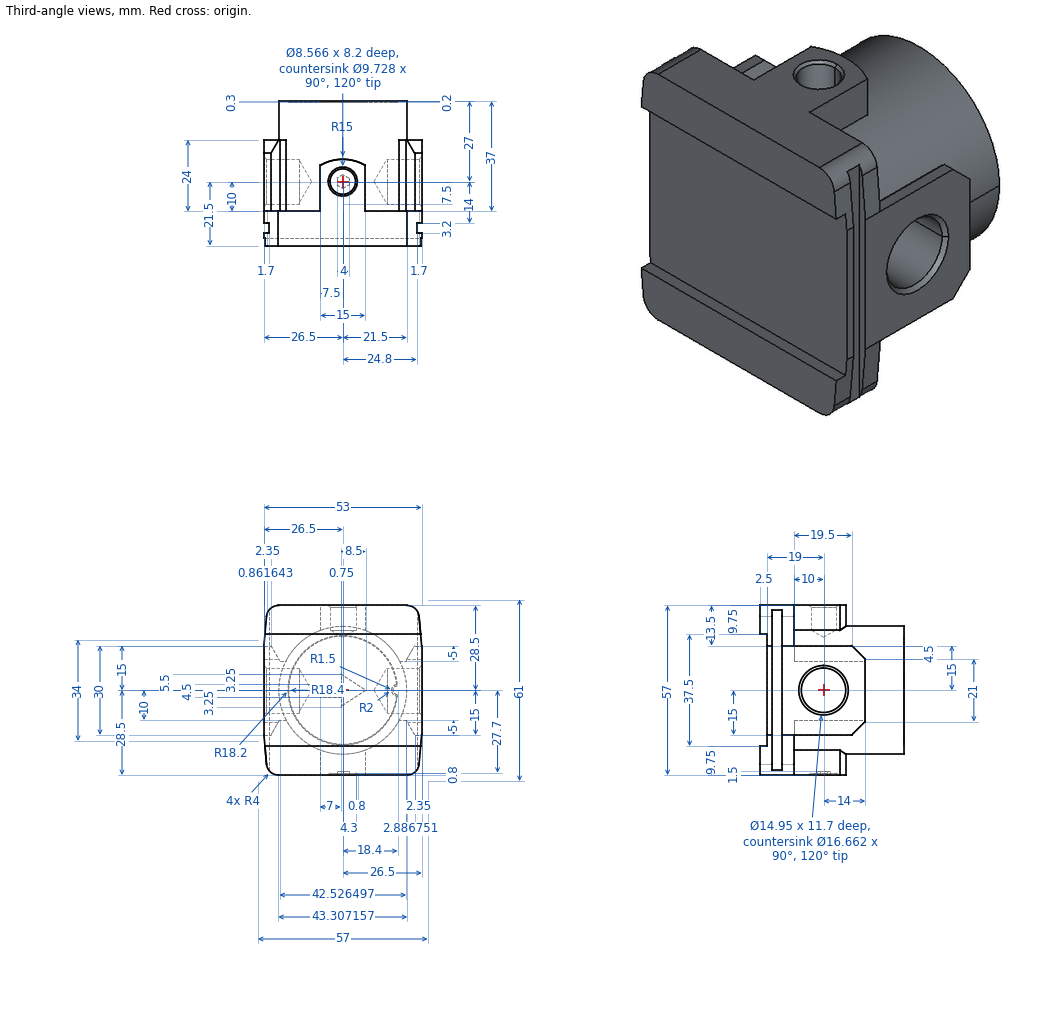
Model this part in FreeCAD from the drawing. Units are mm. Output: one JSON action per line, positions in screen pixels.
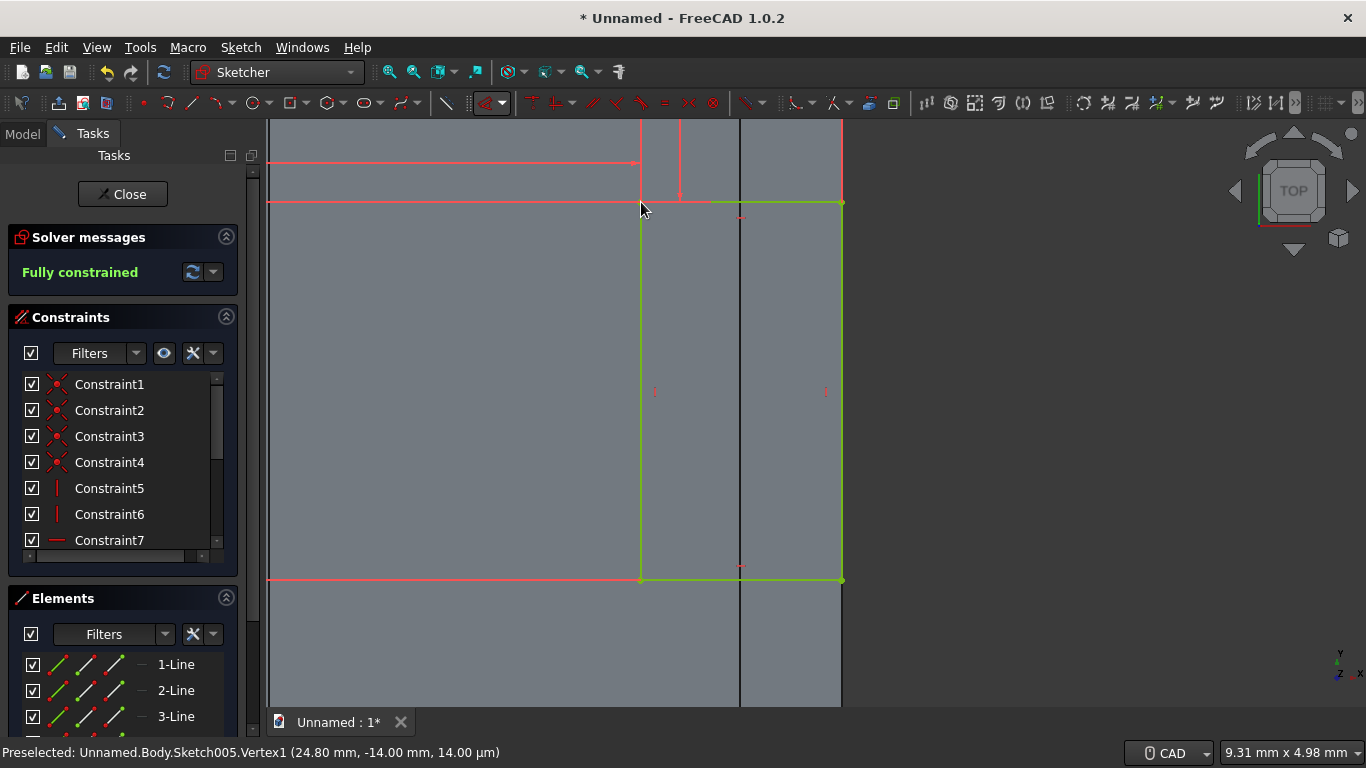
{"action": "left_click", "coordinate": [123, 194]}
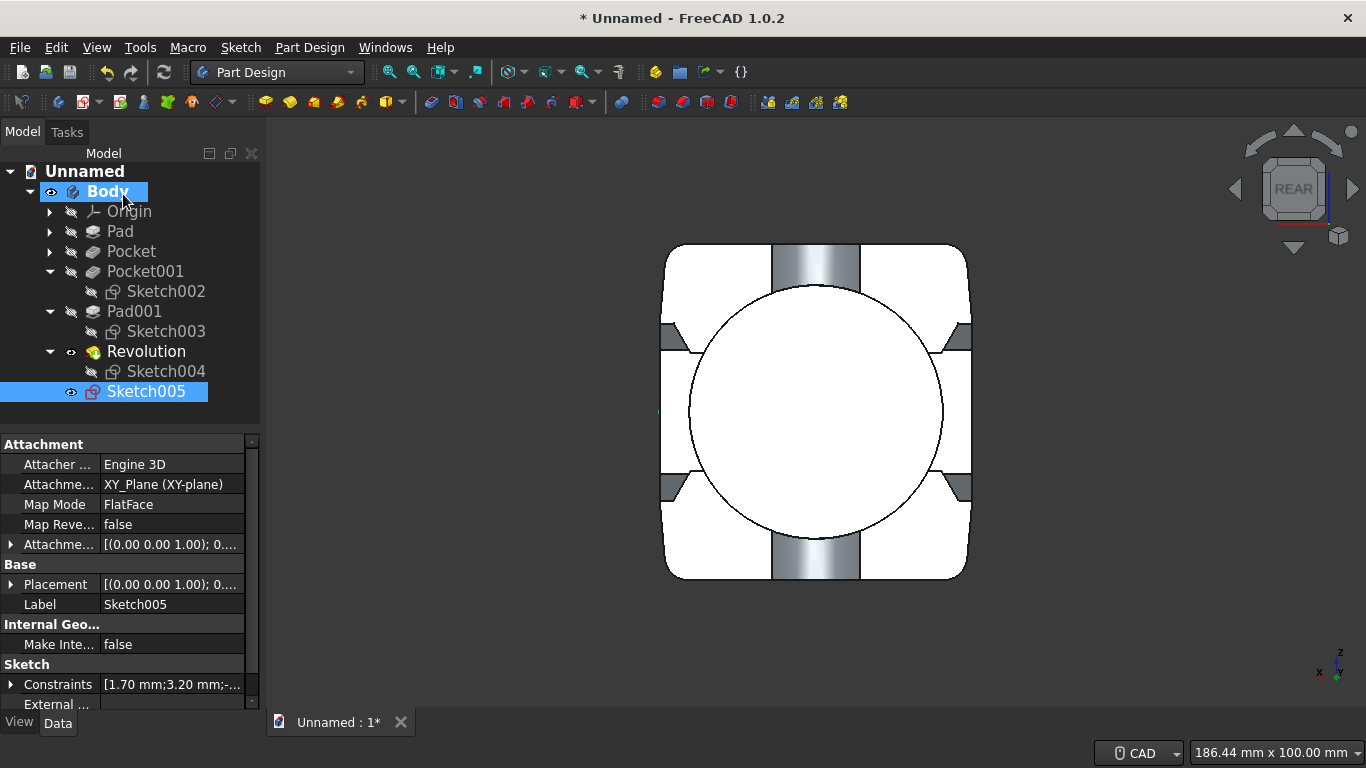
{"action": "left_click", "coordinate": [432, 102]}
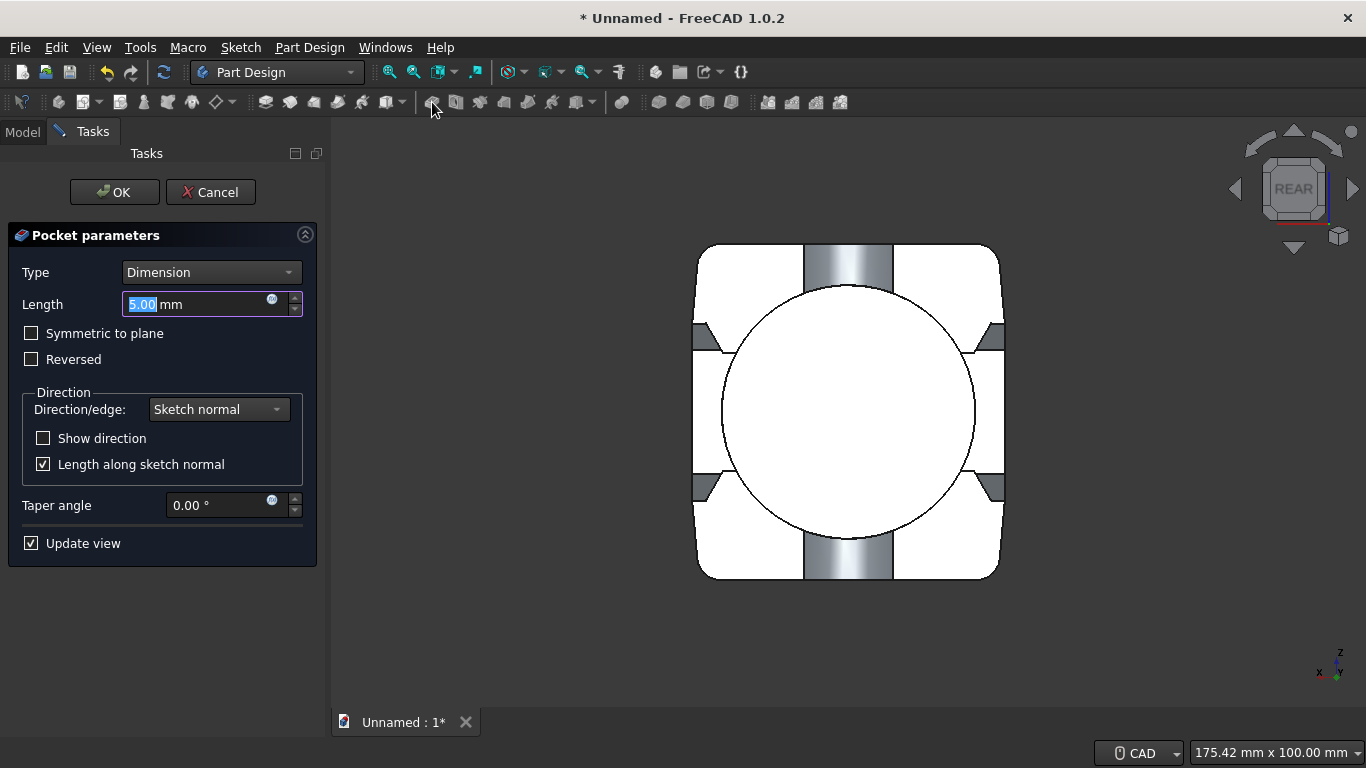
{"action": "type", "text": "57"}
{"action": "key", "text": "Tab"}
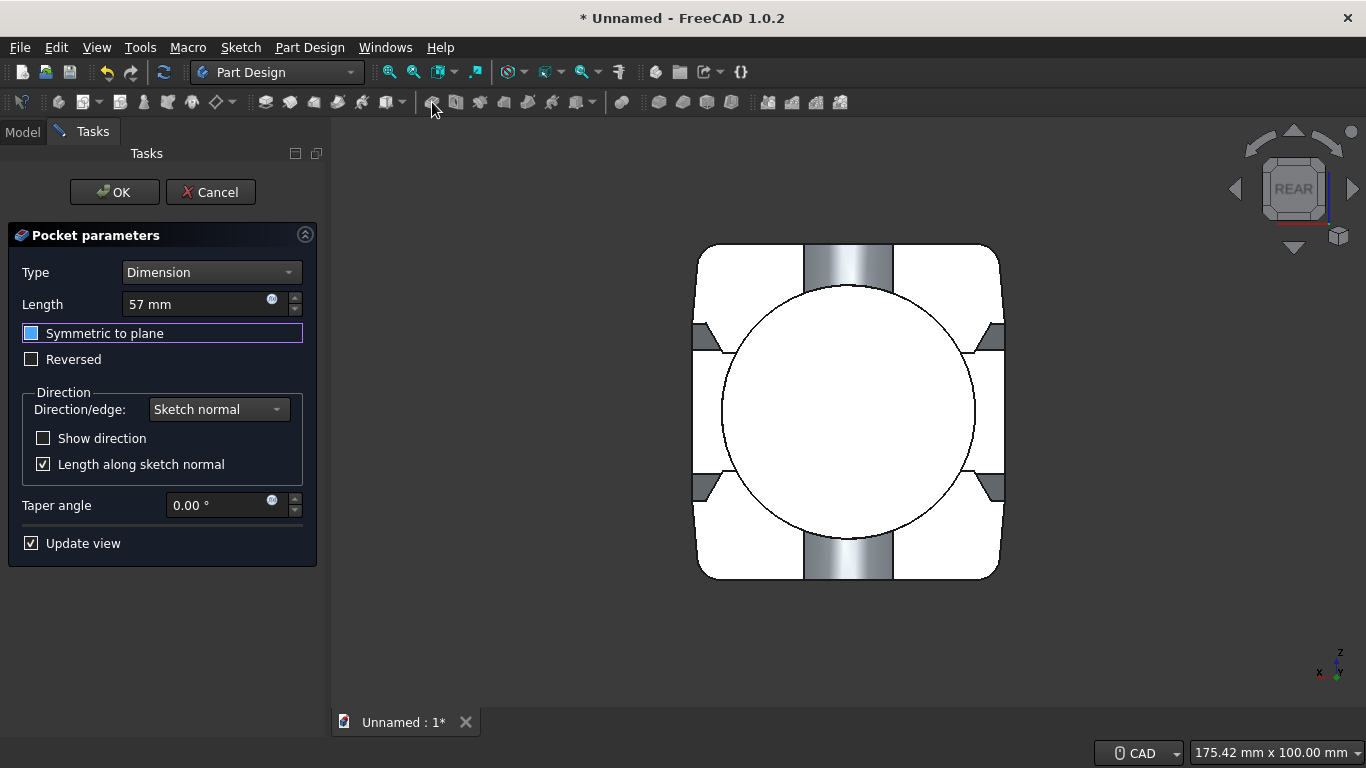
{"action": "left_click", "coordinate": [30, 333]}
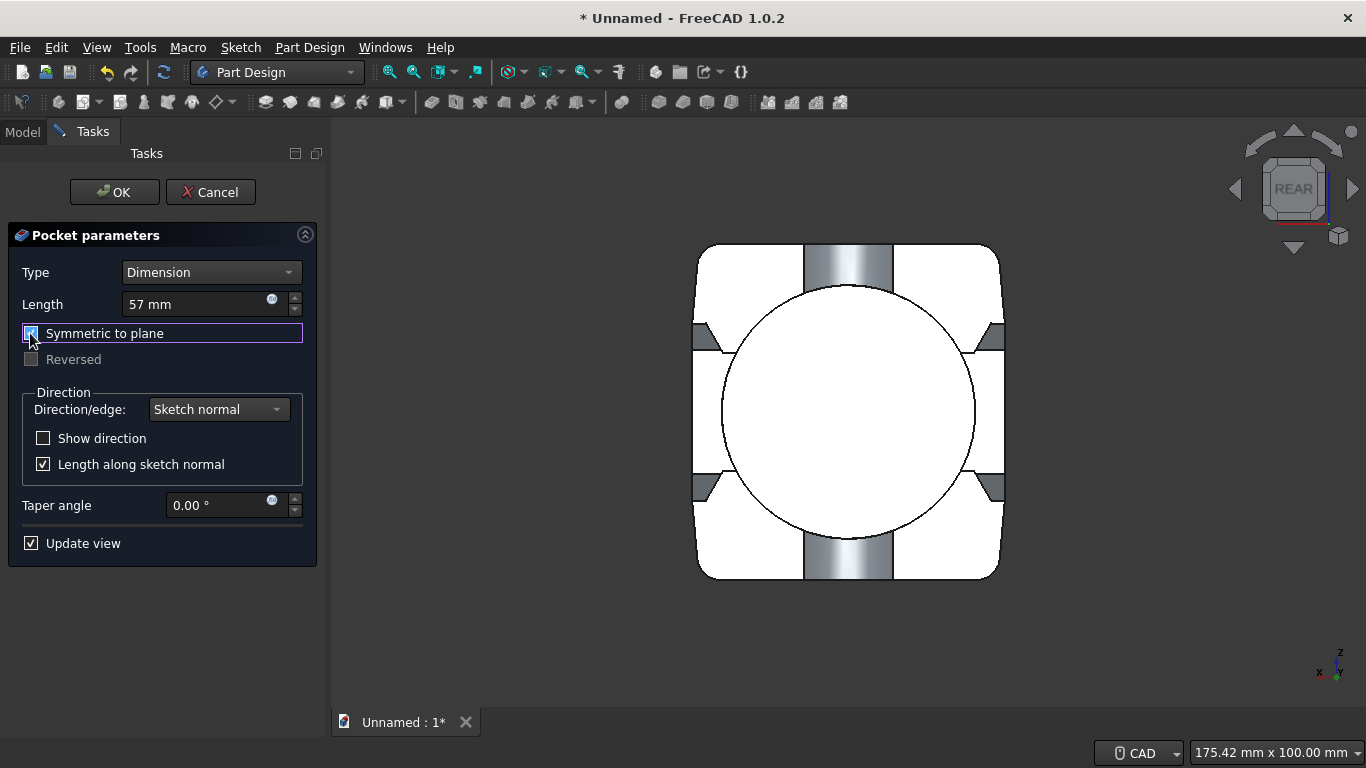
{"action": "left_click", "coordinate": [115, 192]}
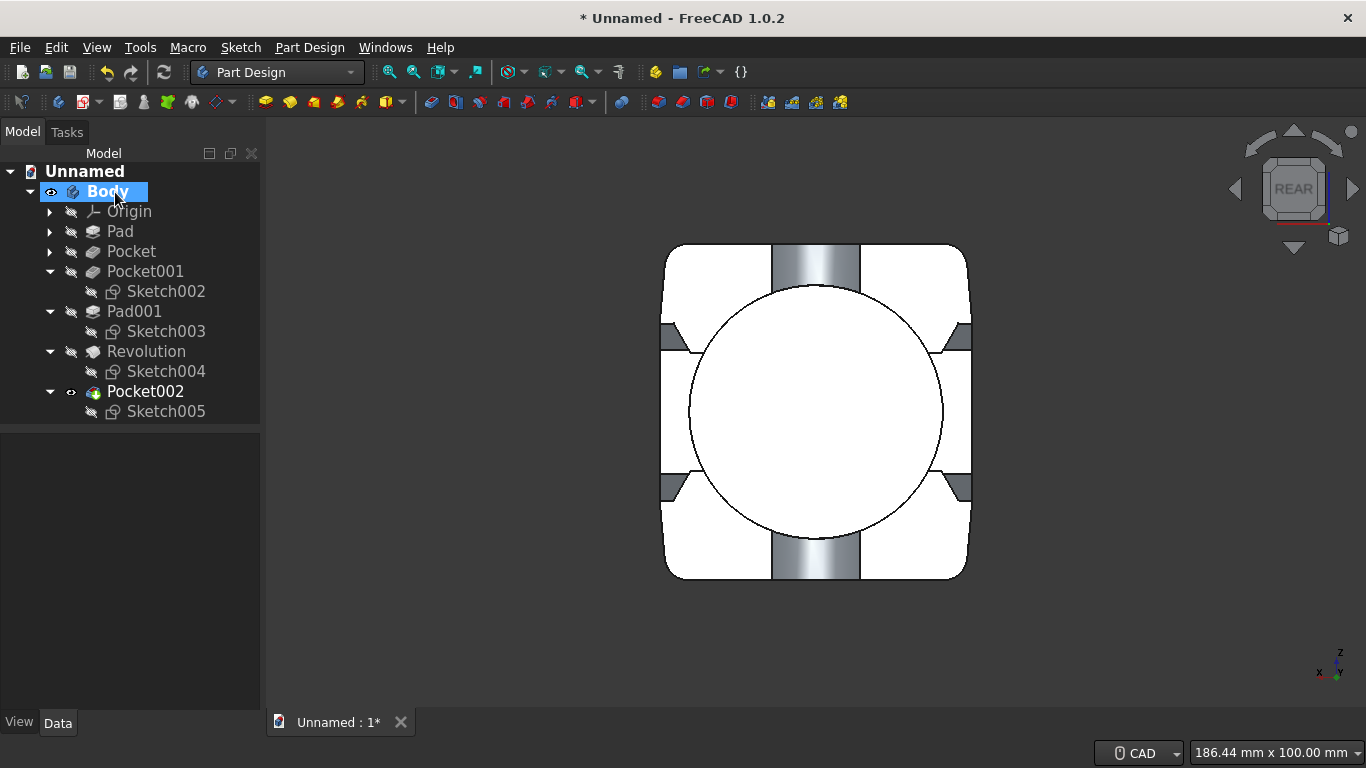
{"action": "left_click", "coordinate": [84, 102]}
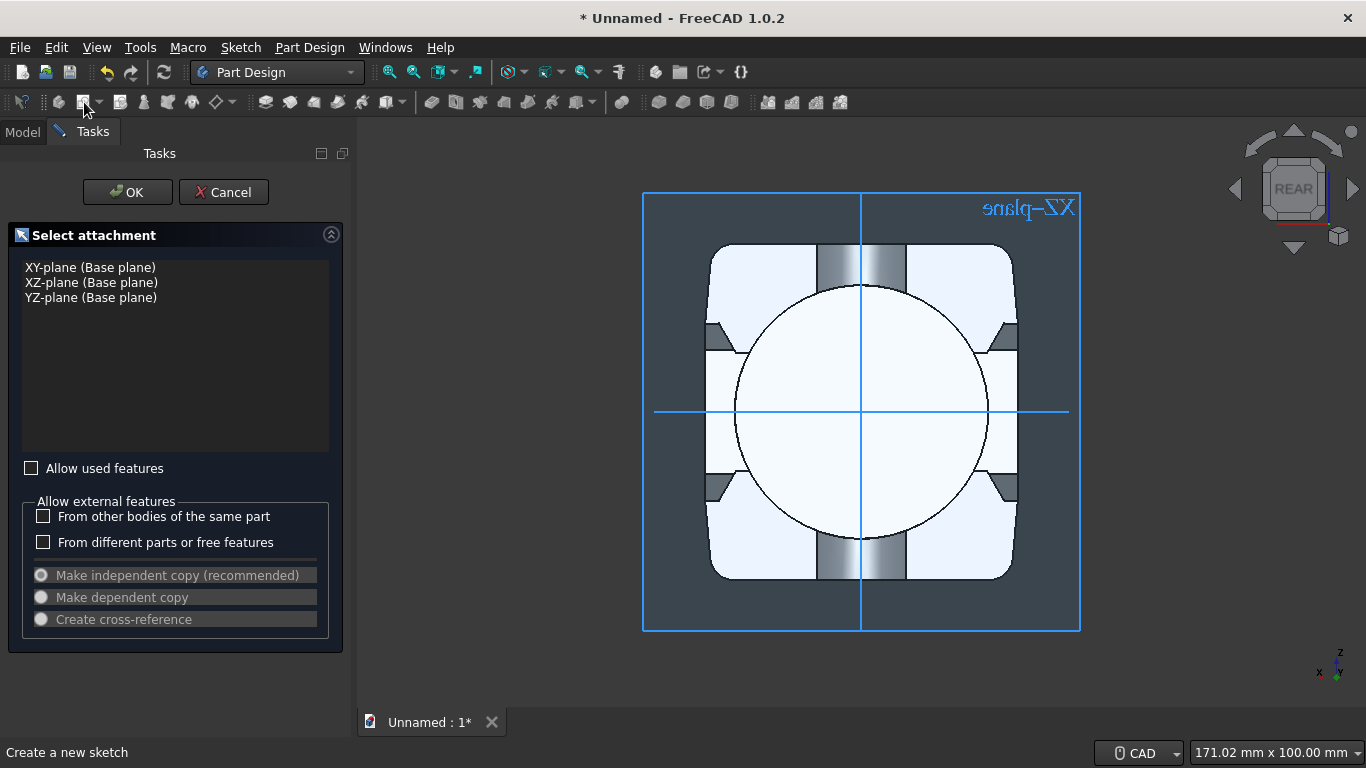
{"action": "left_click", "coordinate": [82, 268]}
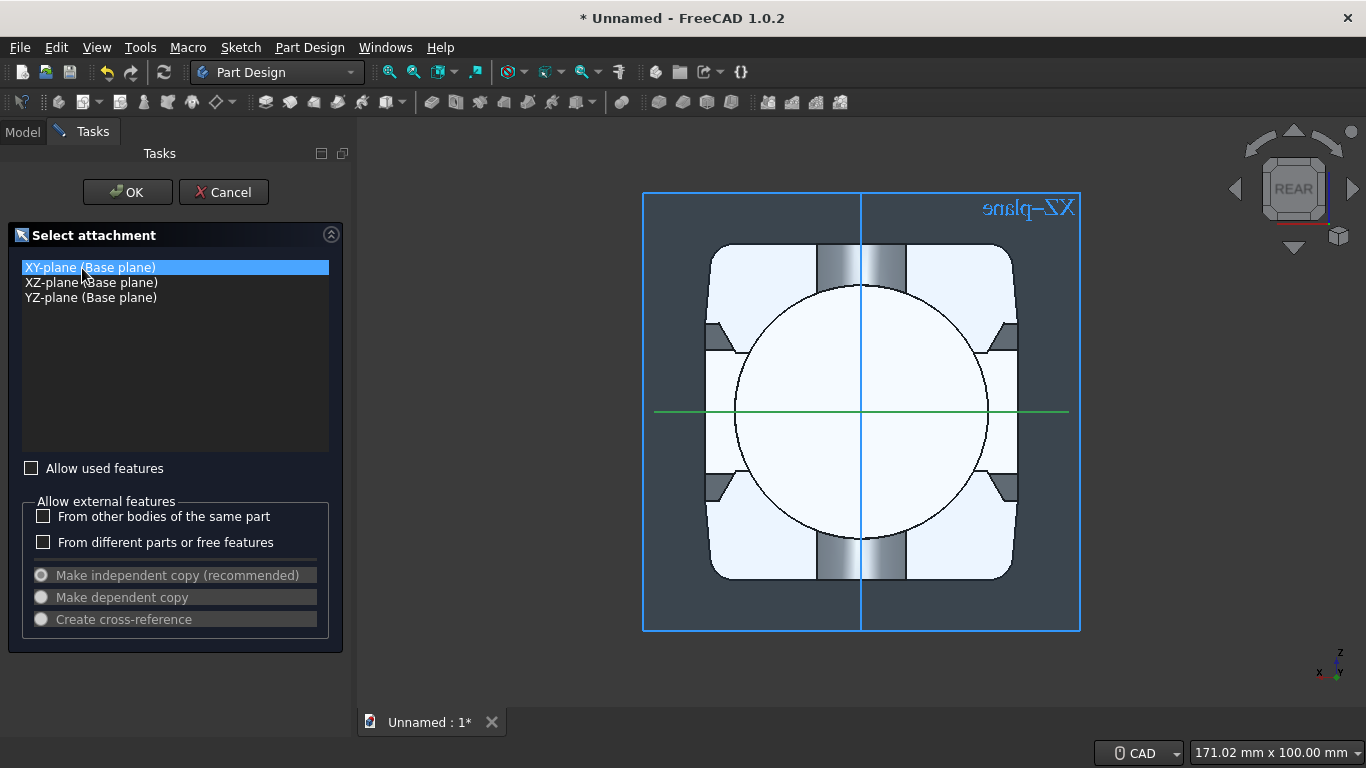
{"action": "left_click", "coordinate": [128, 192]}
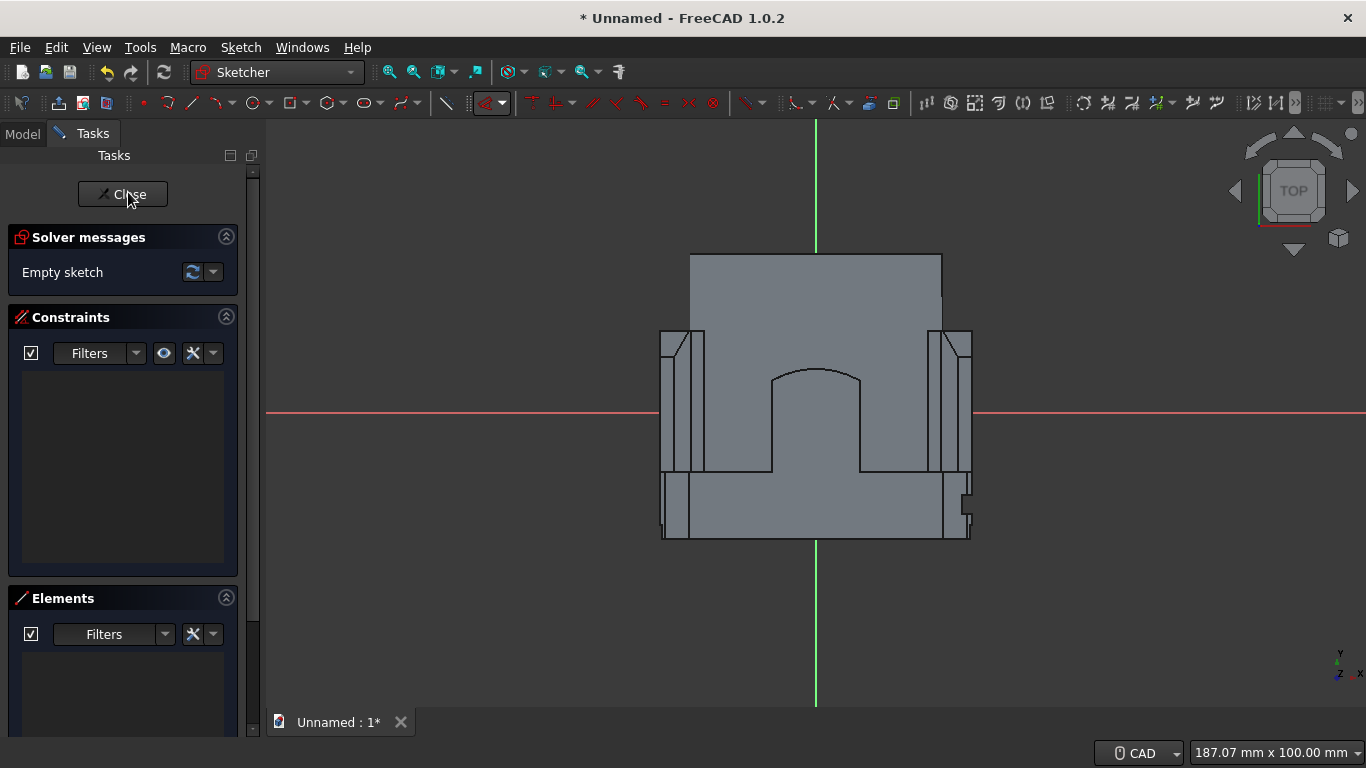
{"action": "left_click", "coordinate": [108, 104]}